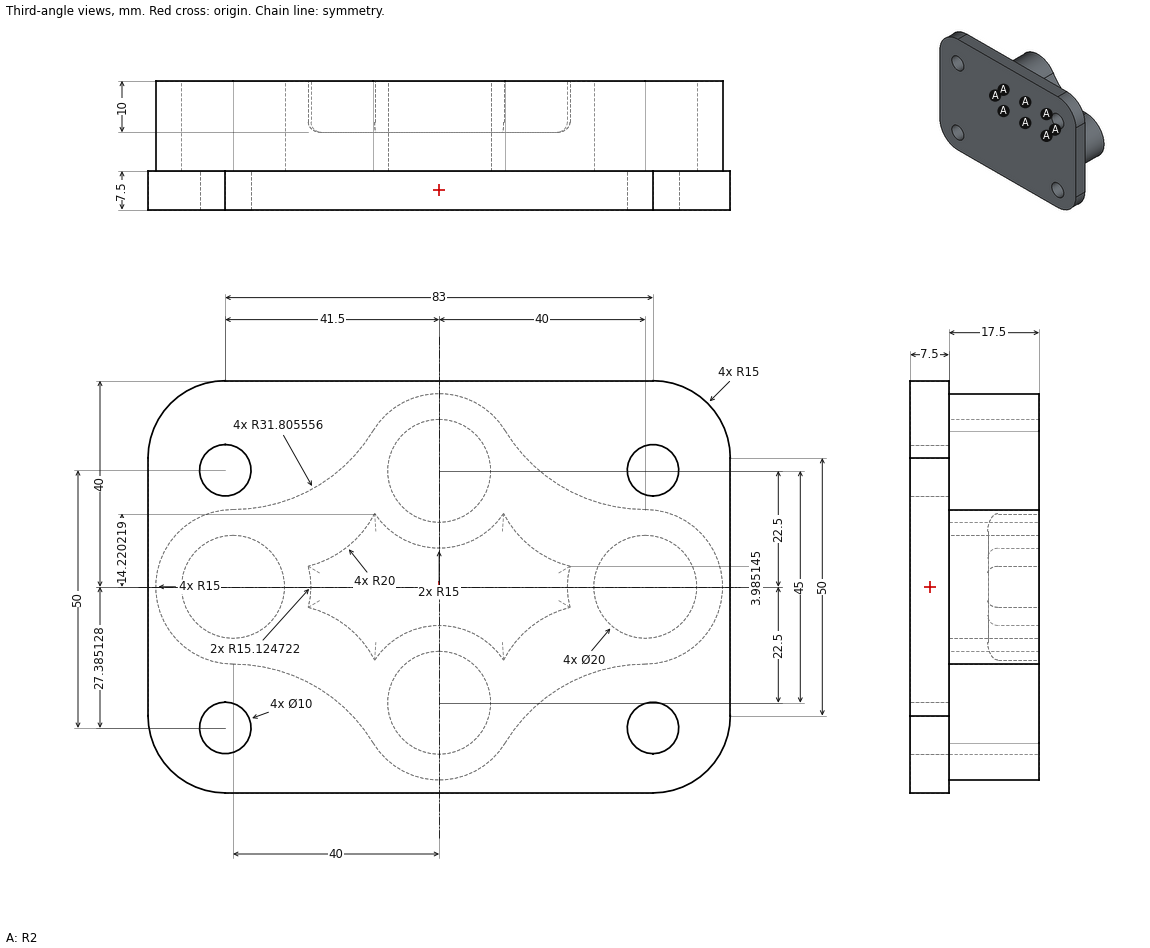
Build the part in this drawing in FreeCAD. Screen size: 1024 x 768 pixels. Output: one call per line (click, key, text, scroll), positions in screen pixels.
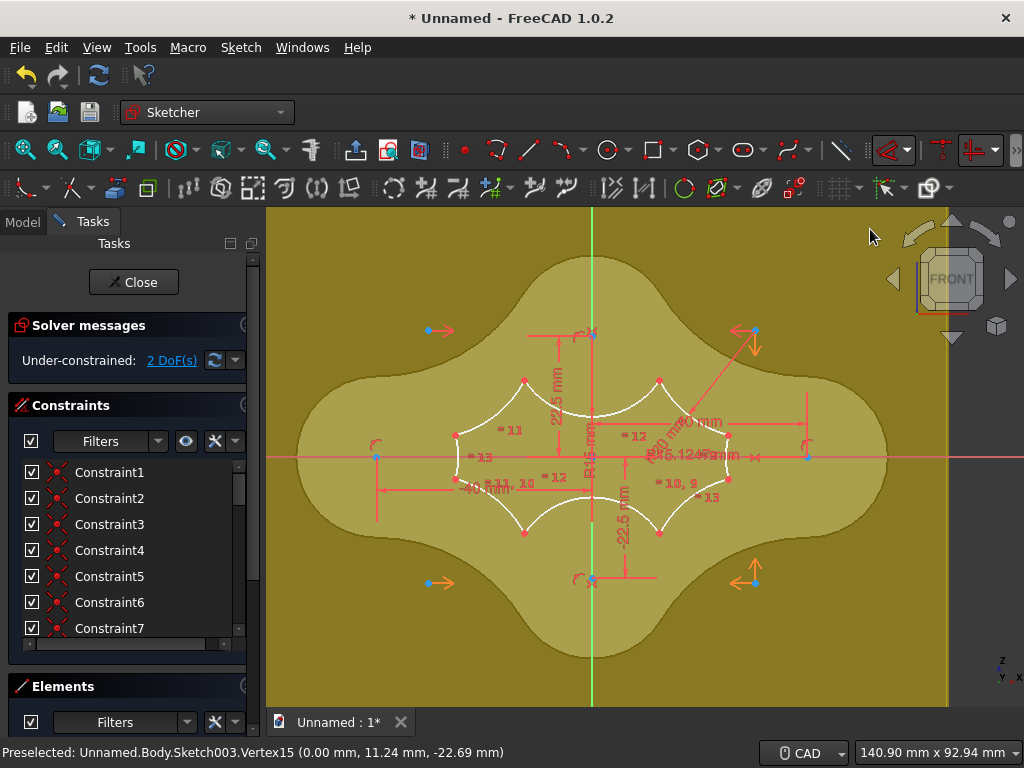
scroll(729, 435, up, 4)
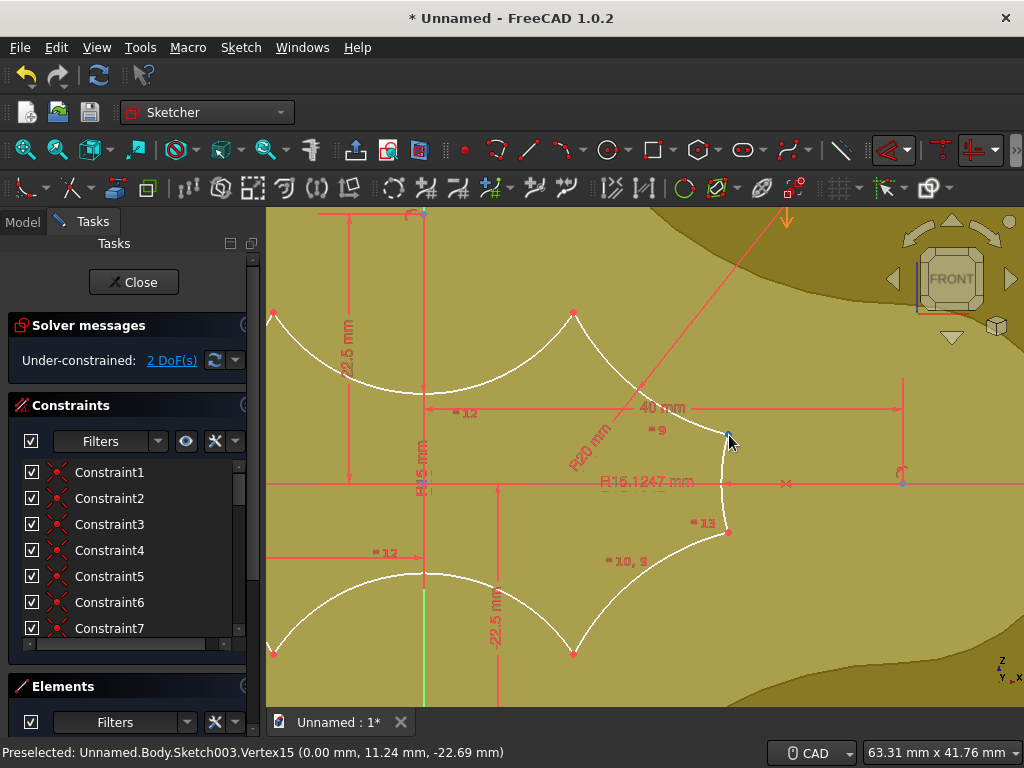
click(728, 435)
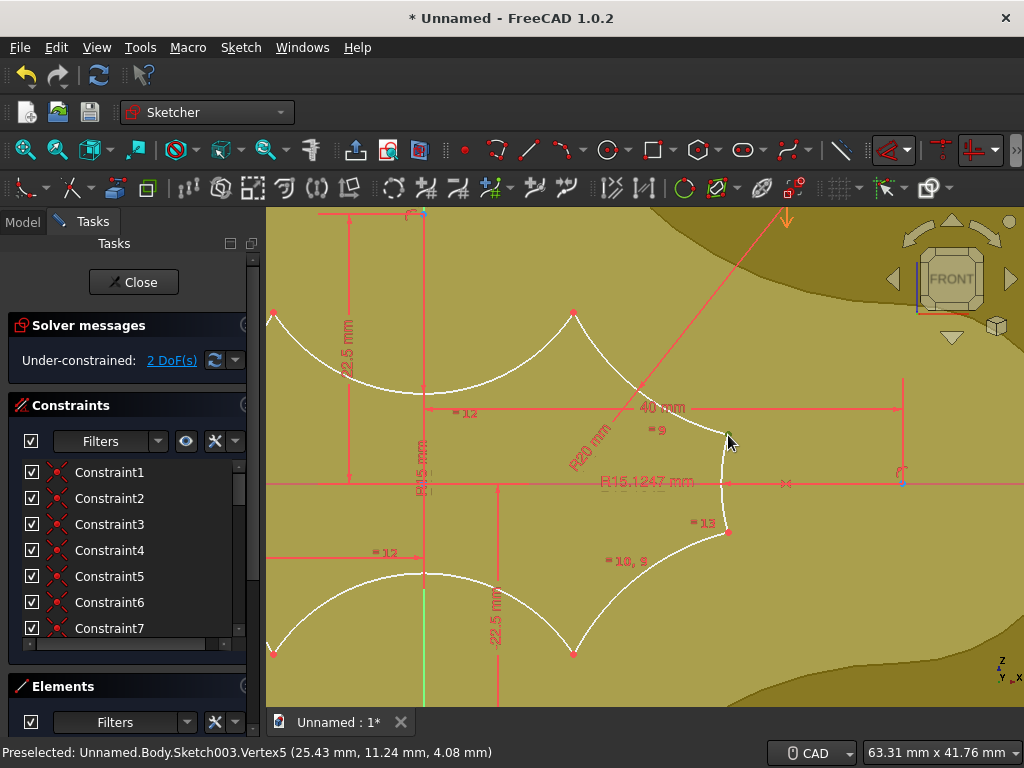
key(i)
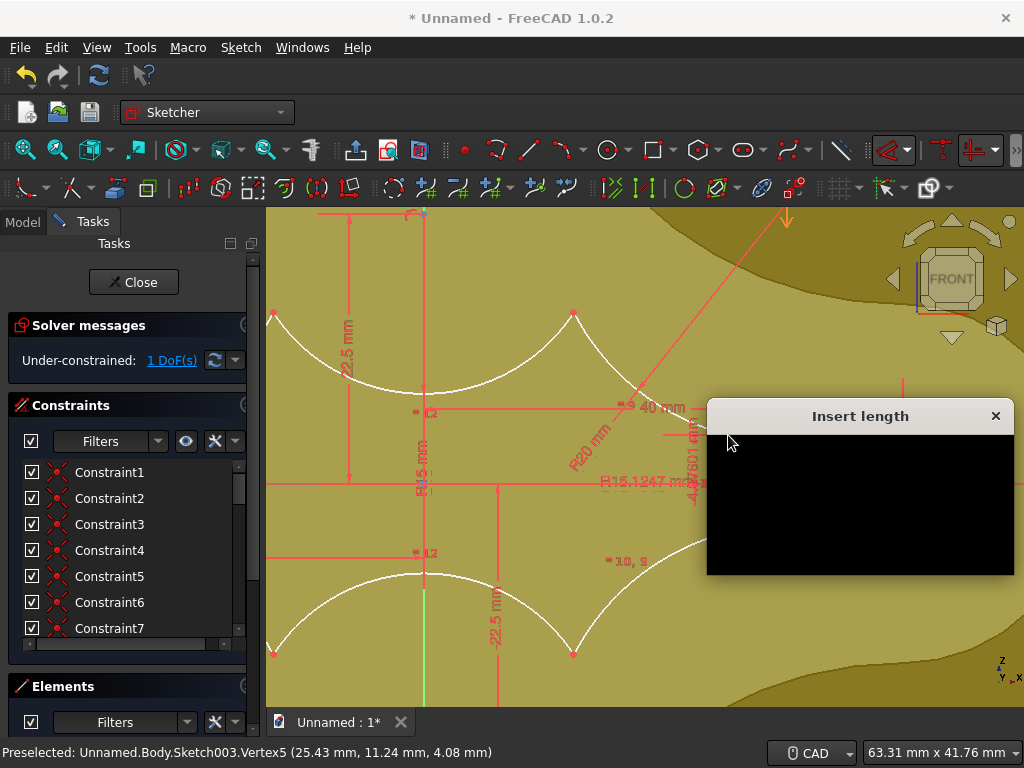
text(3.985145)
key(Return)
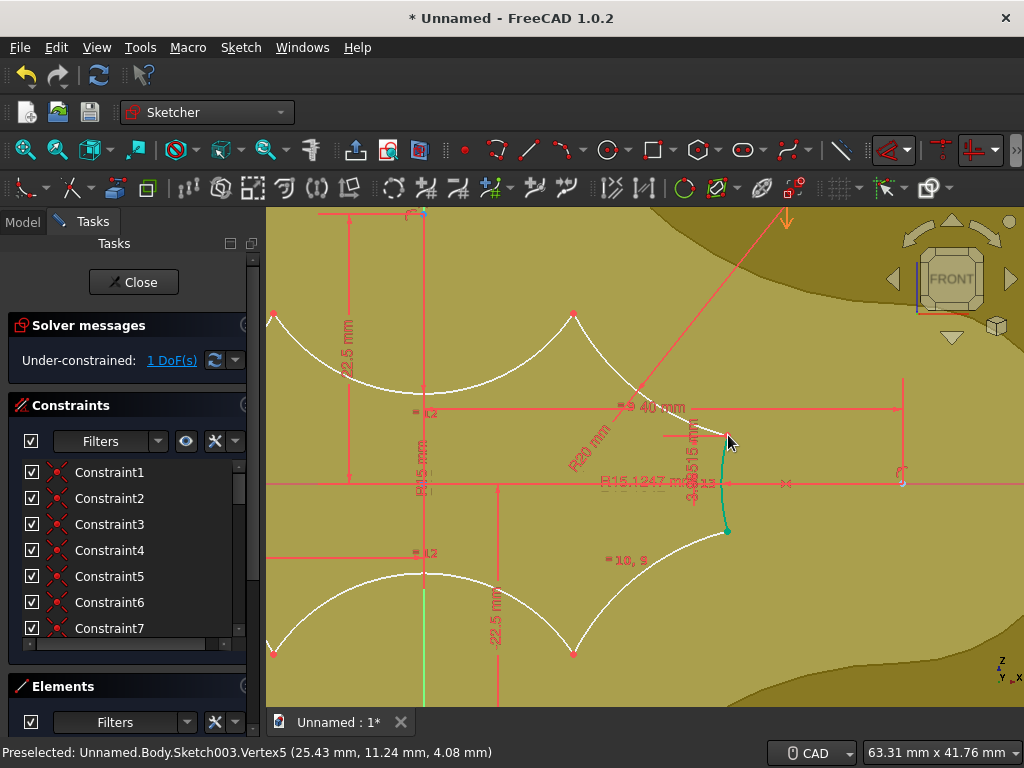
scroll(859, 403, down, 2)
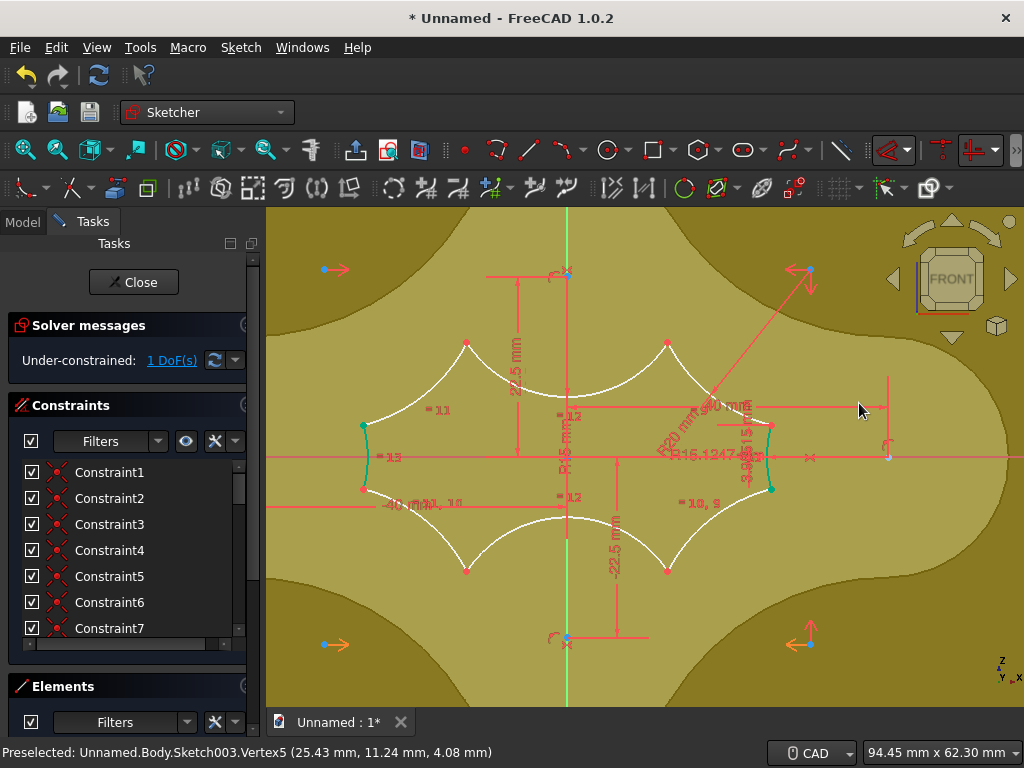
click(467, 343)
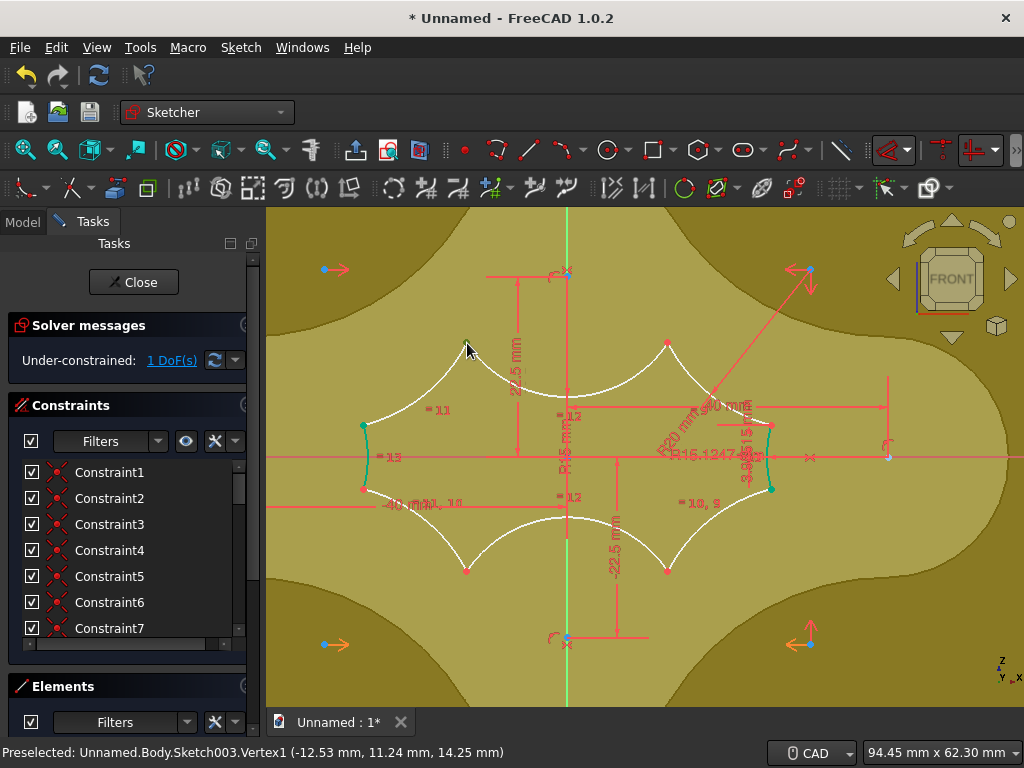
key(i)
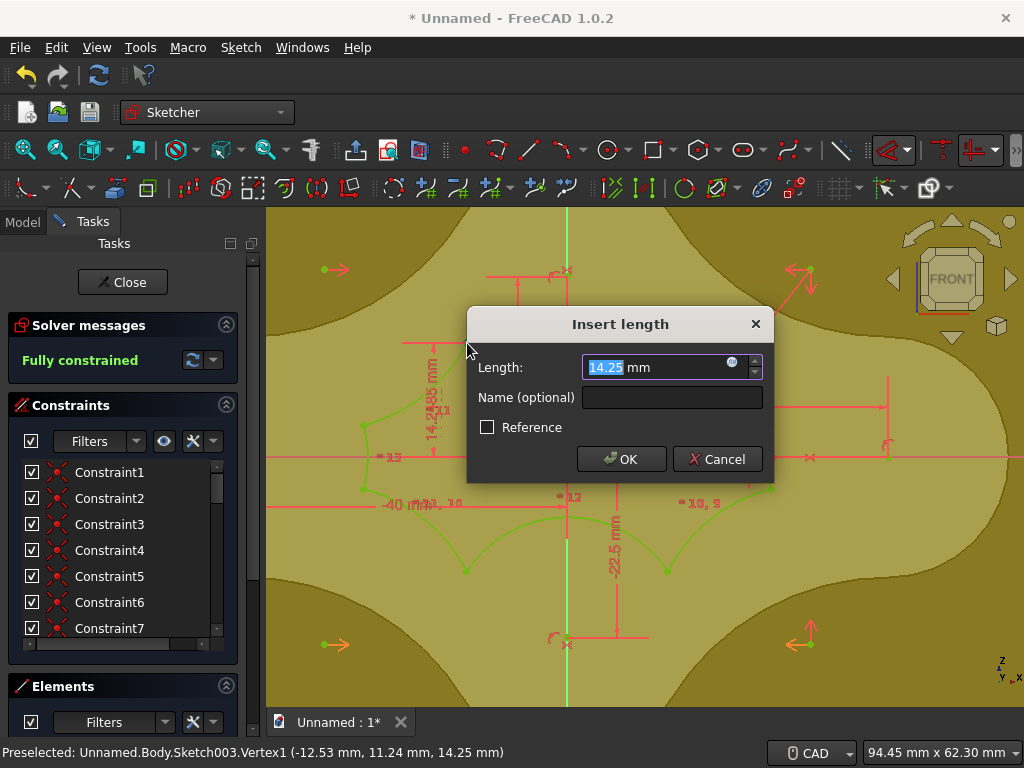
text(14.220219)
key(Return)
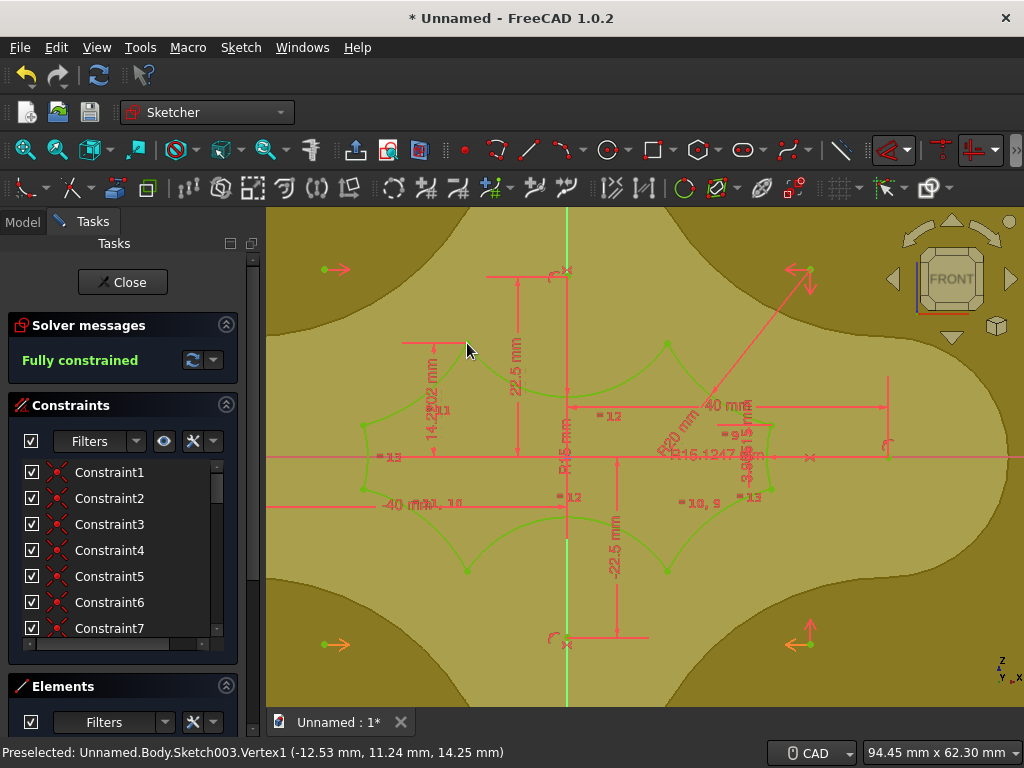
click(123, 282)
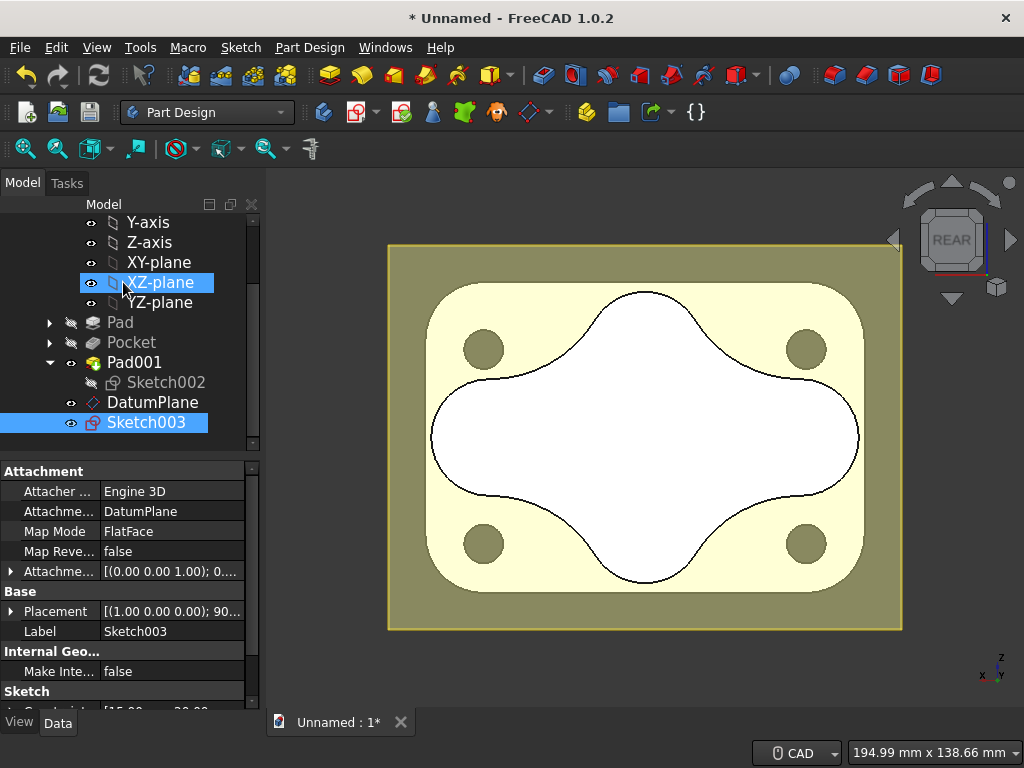
click(544, 76)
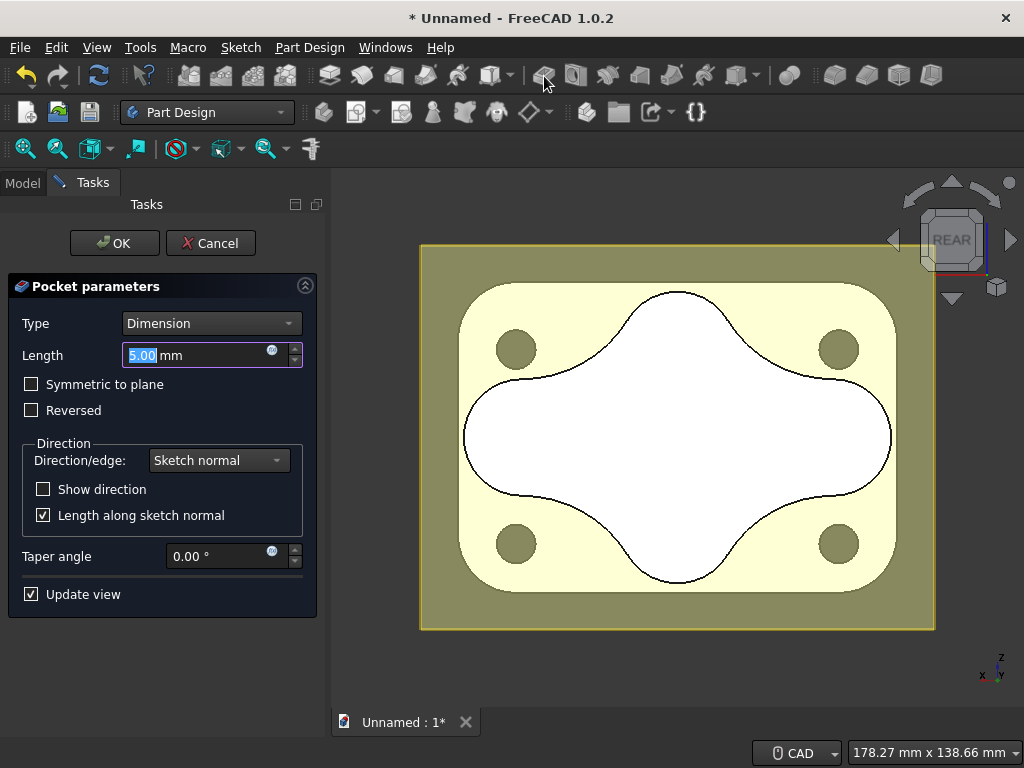
text(10)
key(Tab)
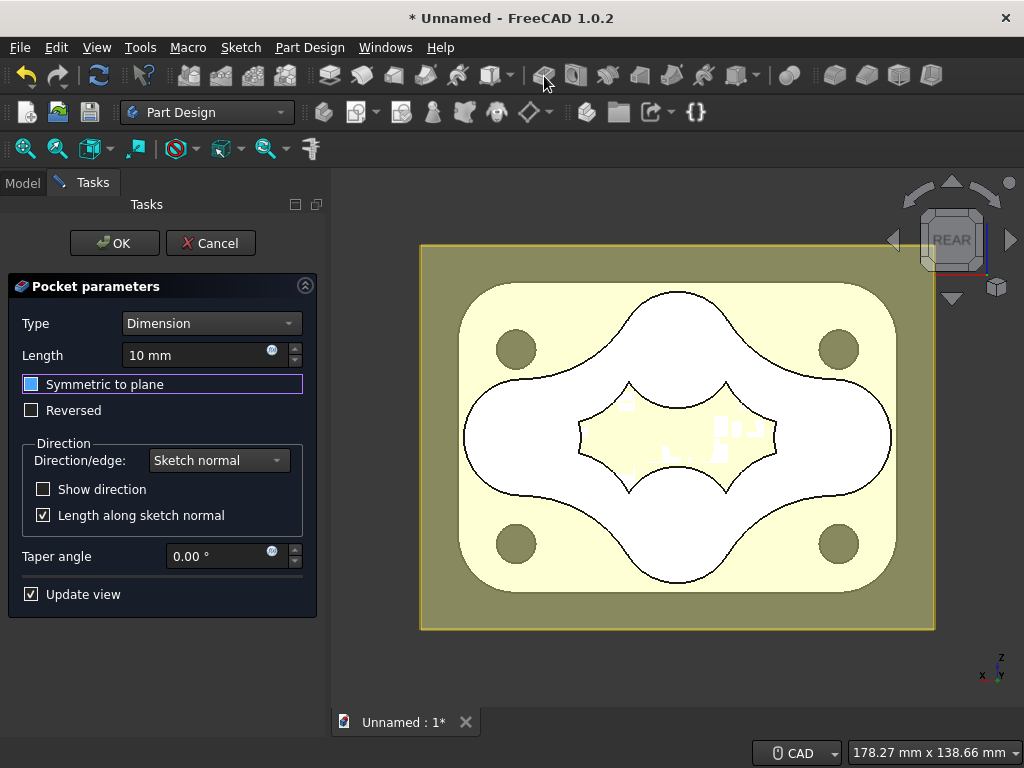
click(115, 243)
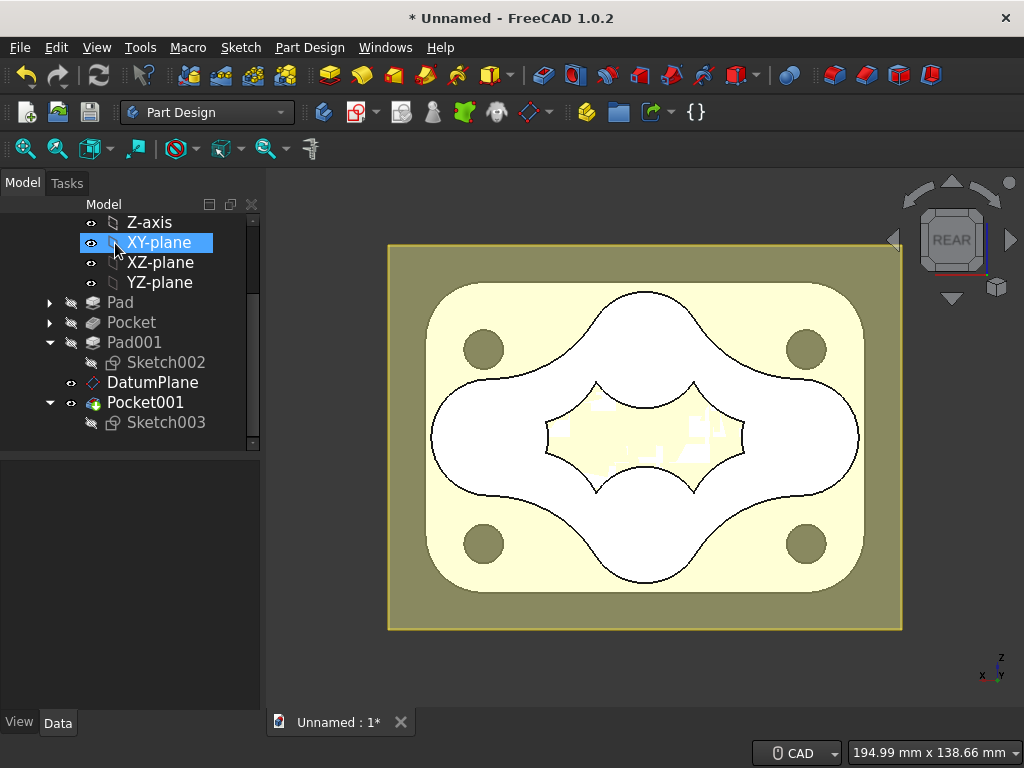
click(116, 383)
key(space)